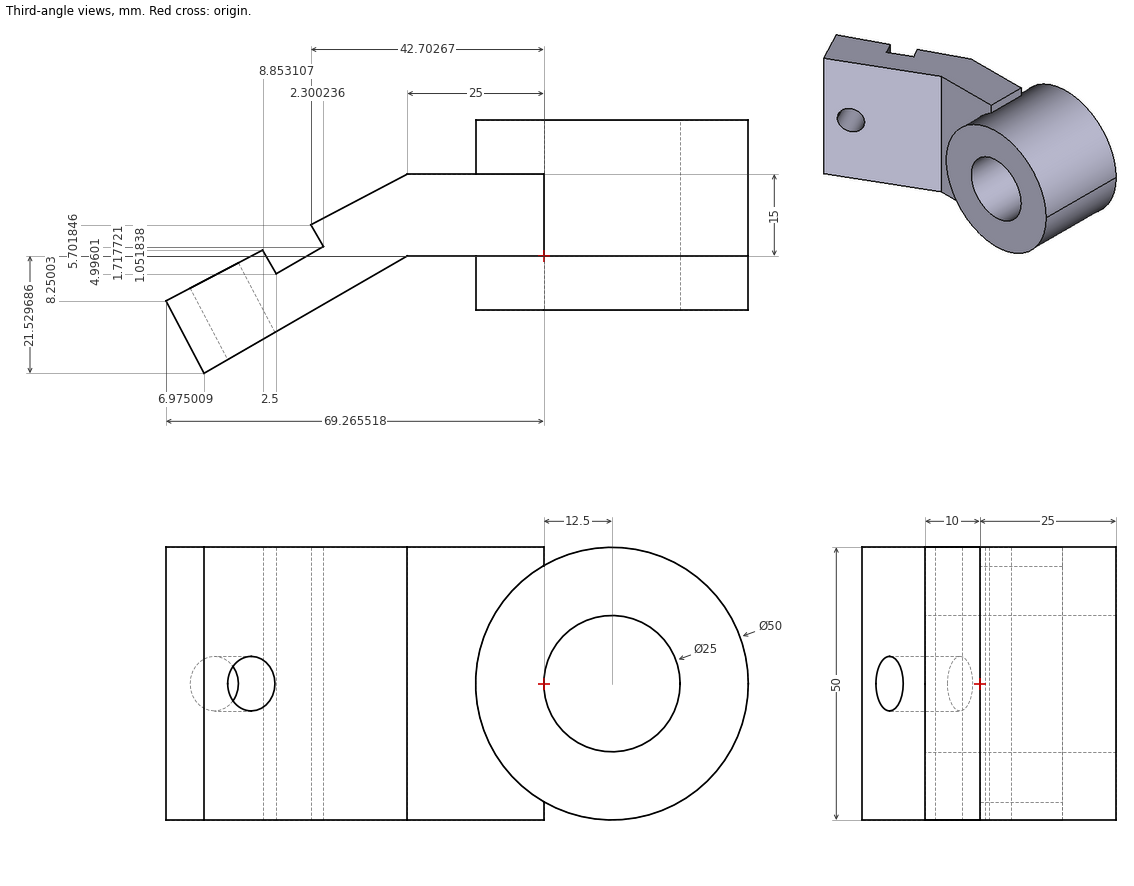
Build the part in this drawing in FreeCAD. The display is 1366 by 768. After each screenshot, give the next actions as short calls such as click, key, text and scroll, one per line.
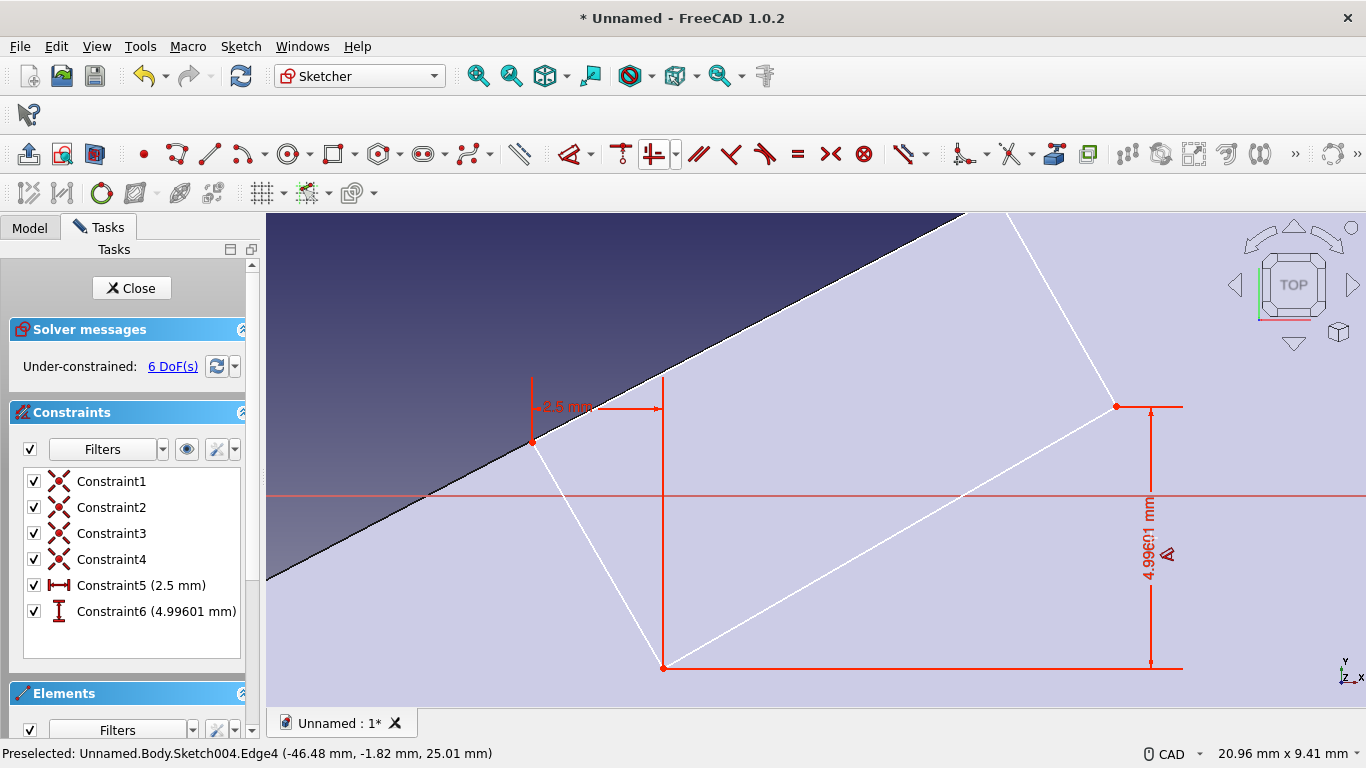
click(1117, 407)
click(1083, 451)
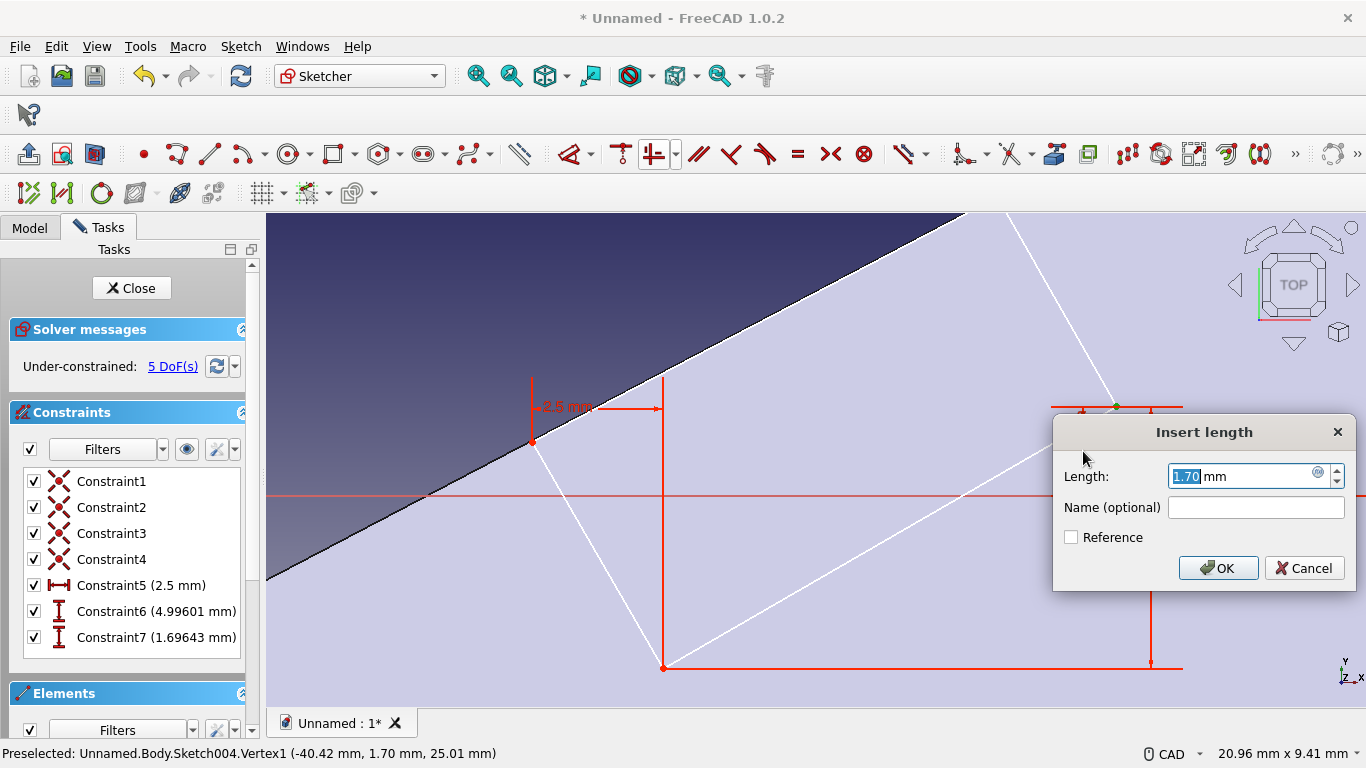
text(1.717721)
key(Return)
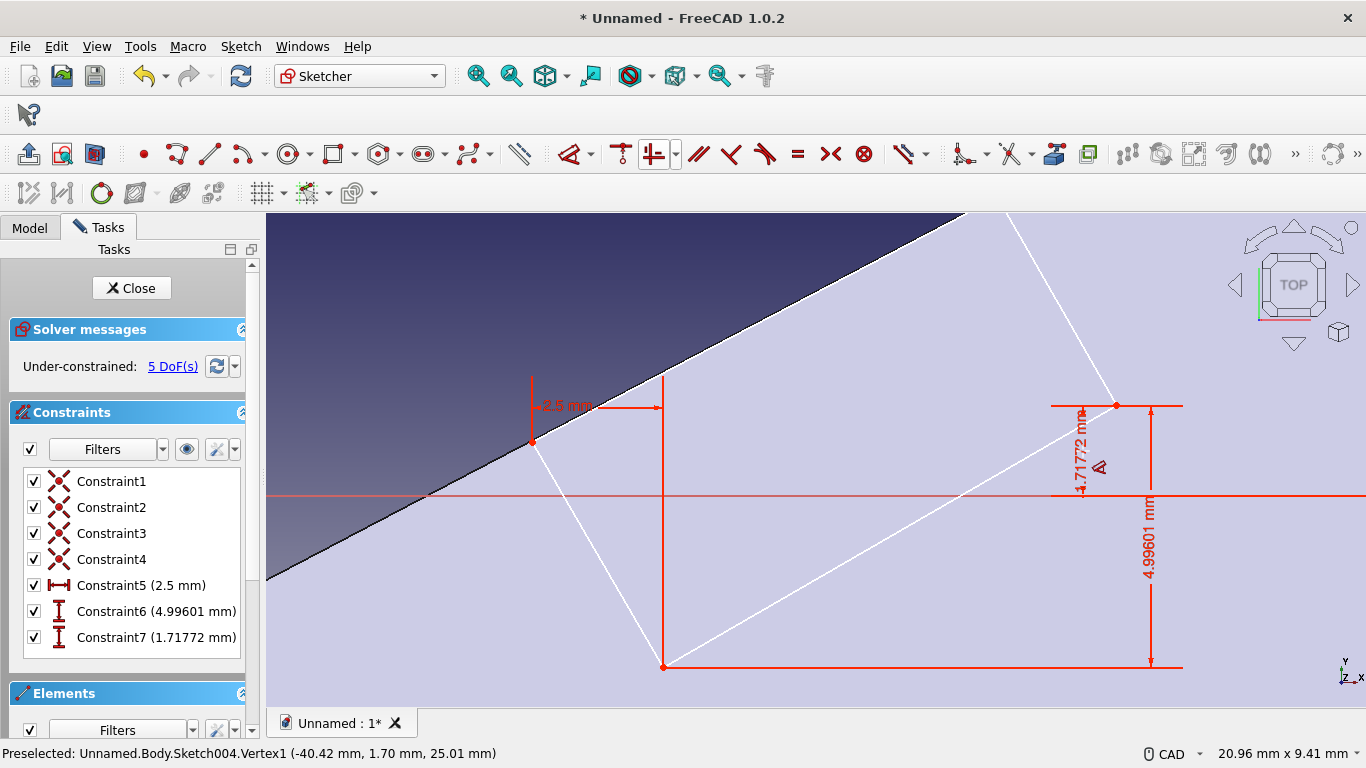
scroll(590, 517, down, 2)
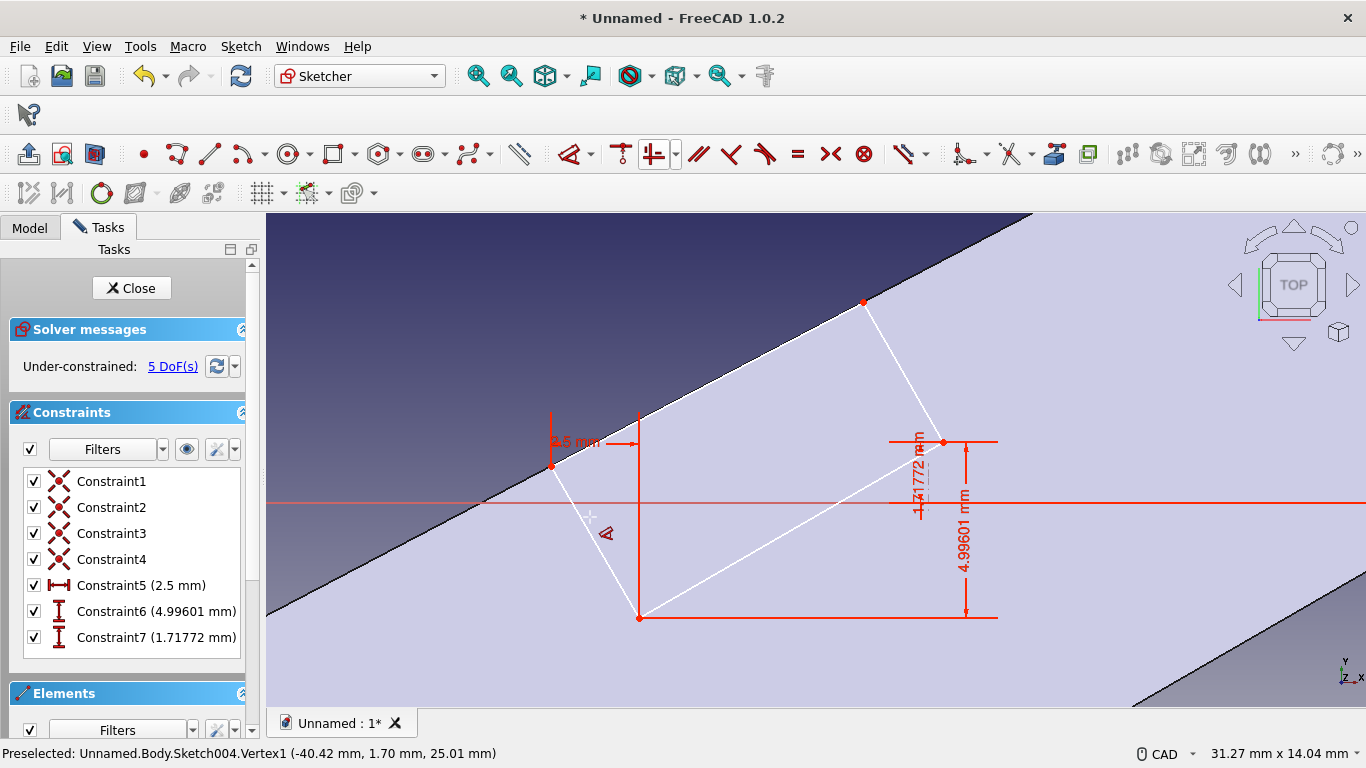
click(863, 303)
click(1032, 269)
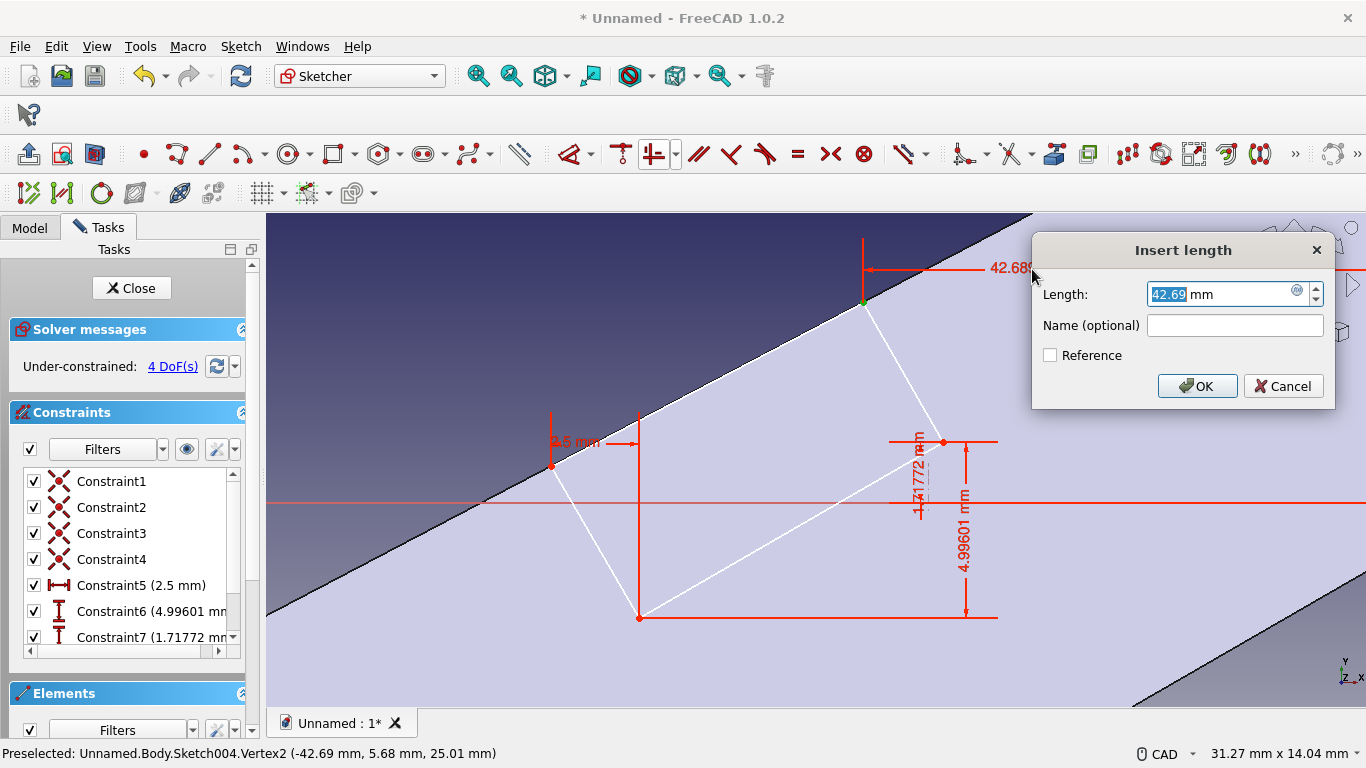
text(42.70267)
key(Return)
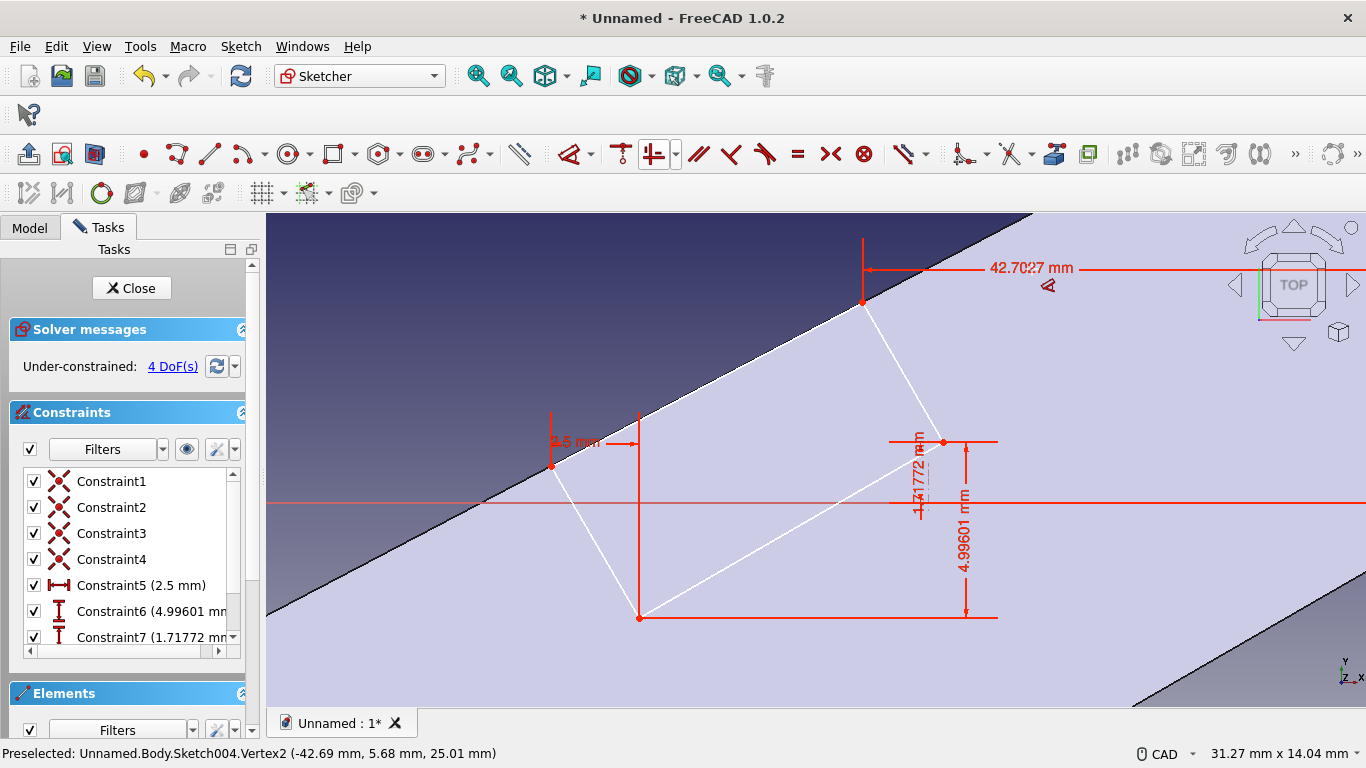
click(863, 303)
click(829, 403)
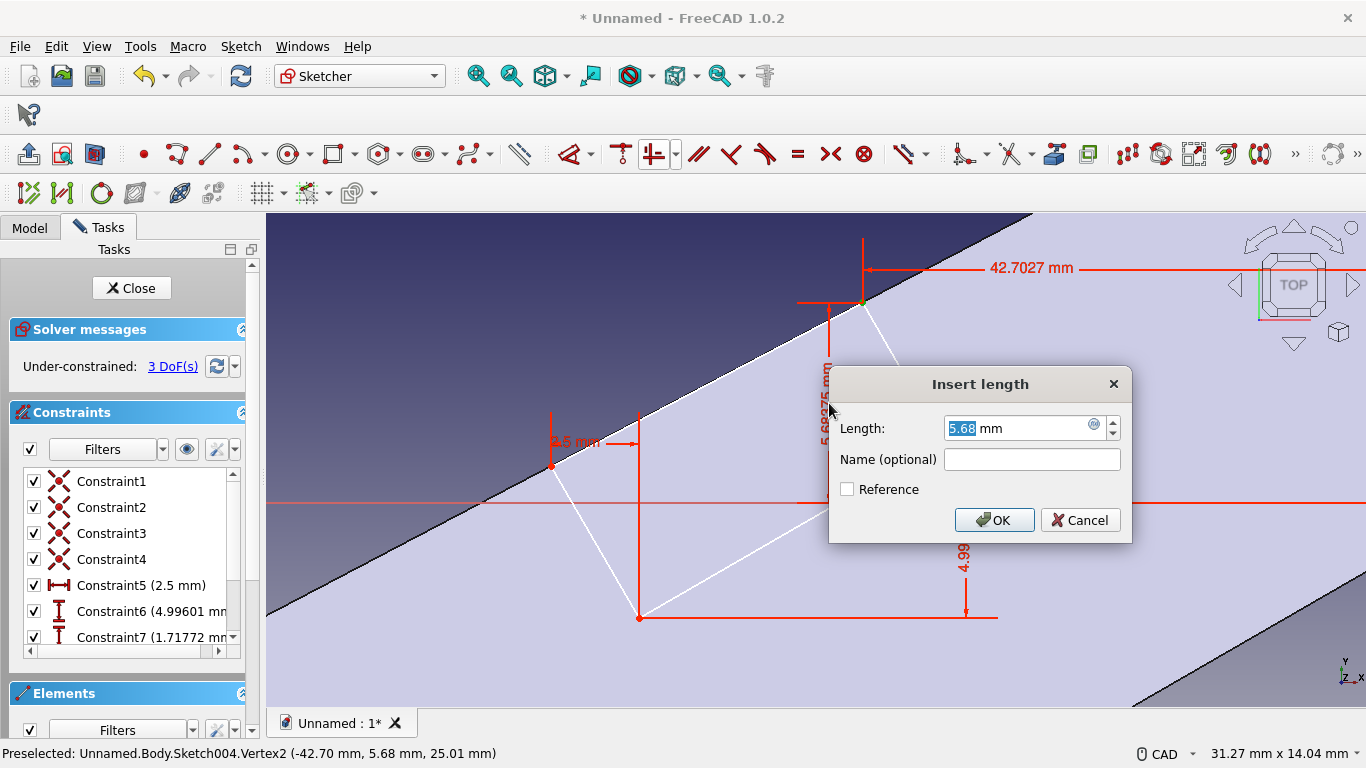
text(5.701846)
key(Return)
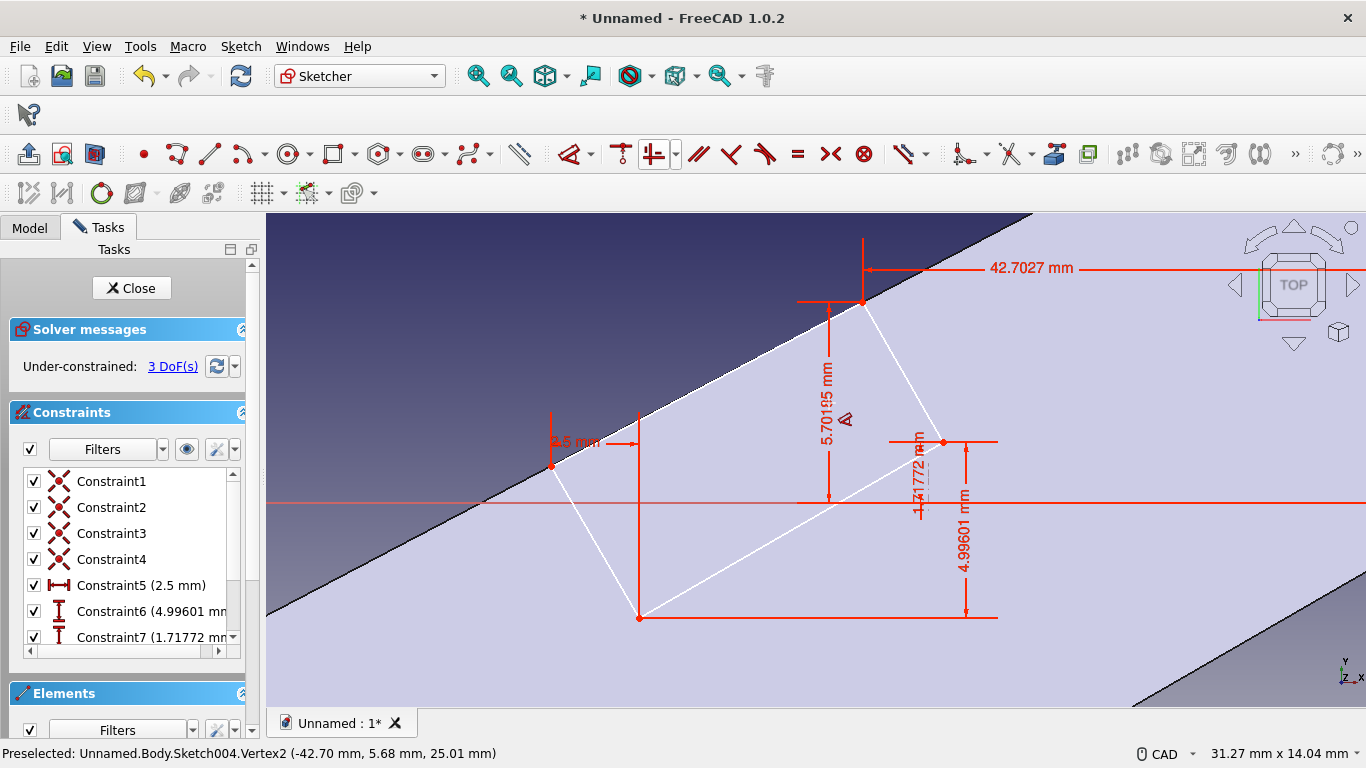
click(551, 467)
click(517, 485)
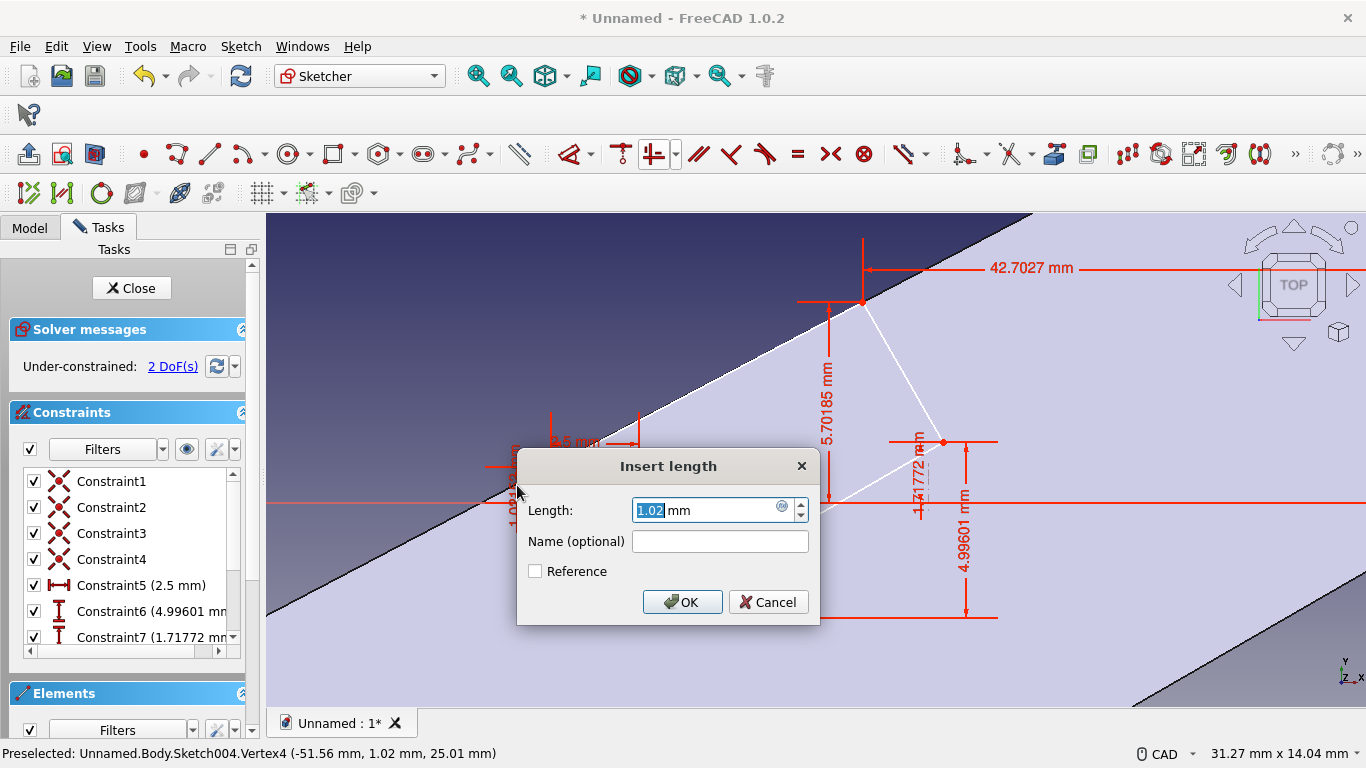
text(1.051838)
key(Return)